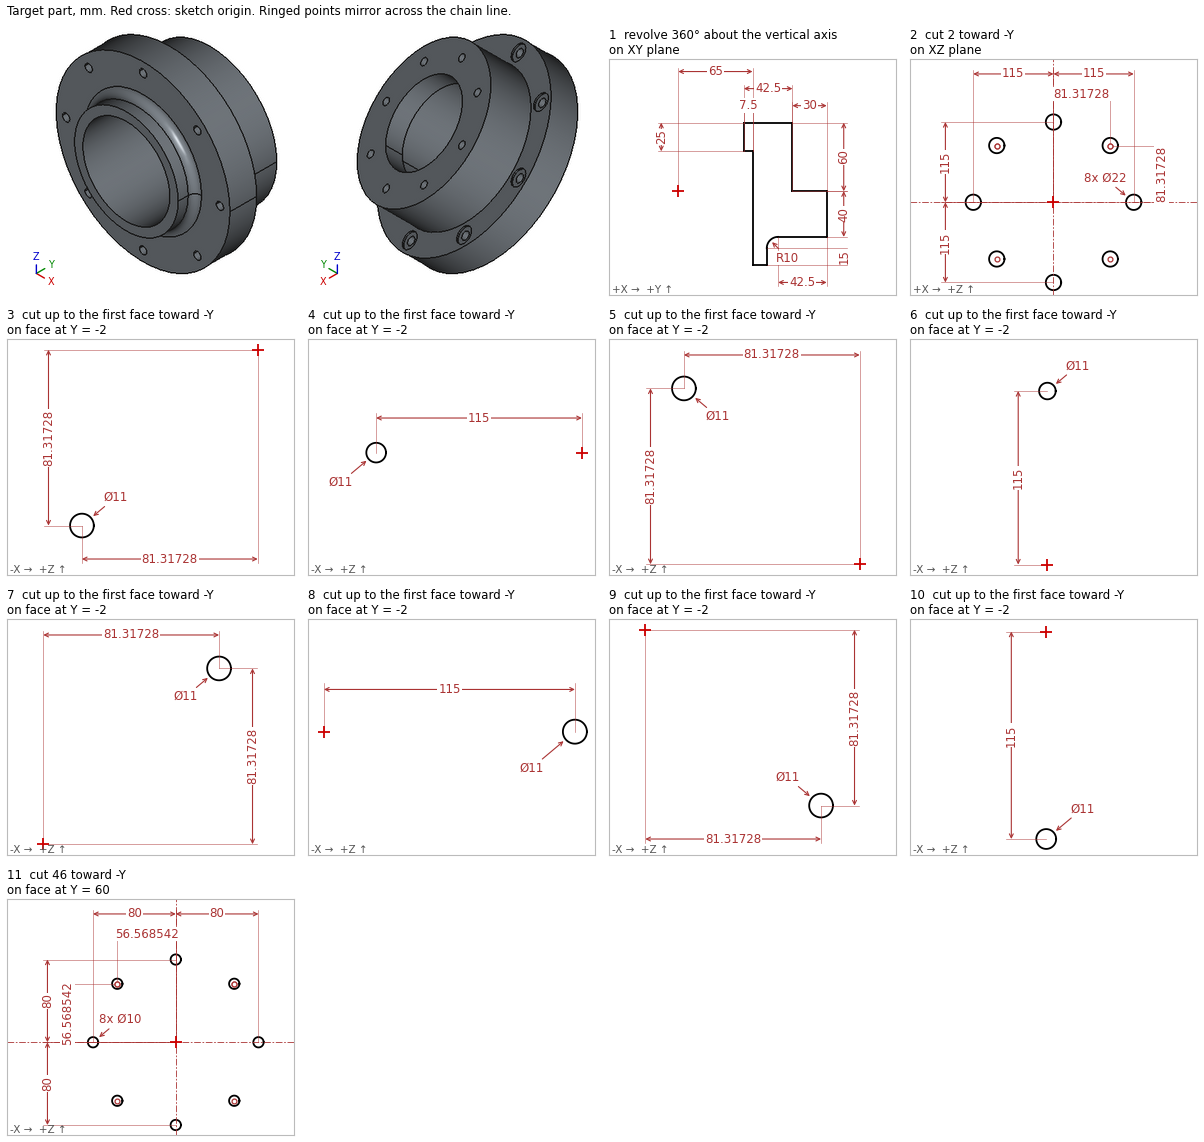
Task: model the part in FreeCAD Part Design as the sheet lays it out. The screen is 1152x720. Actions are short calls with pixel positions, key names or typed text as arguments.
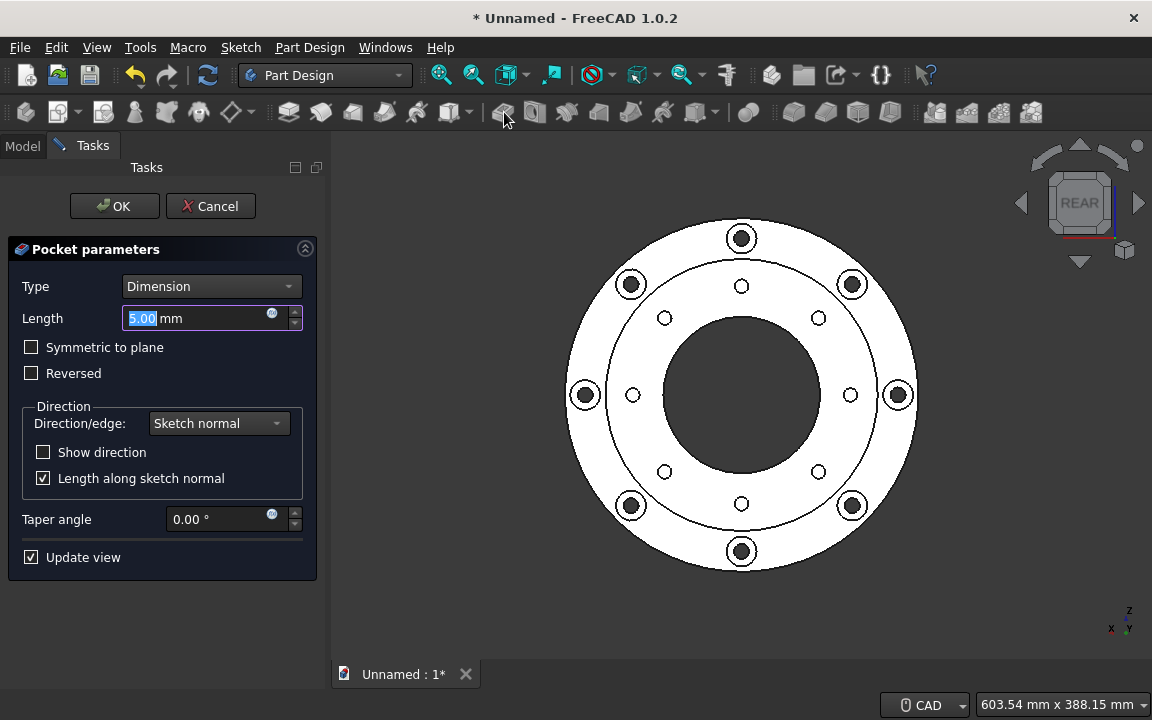
text(46)
key(Tab)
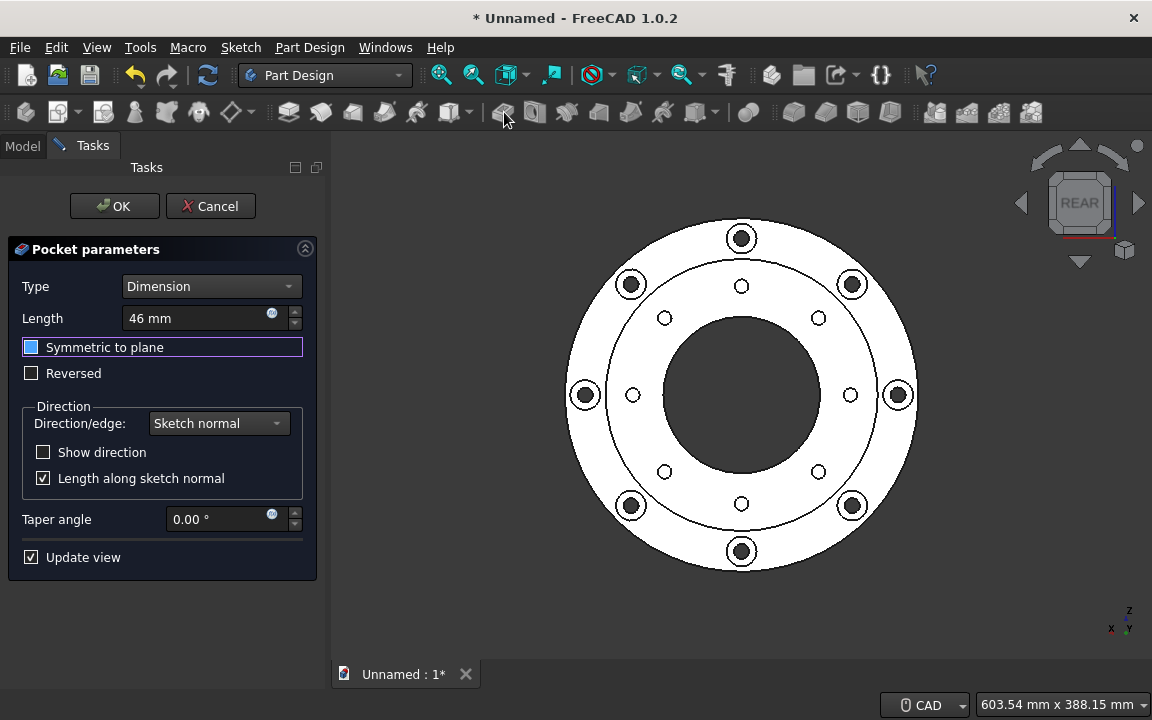
click(115, 206)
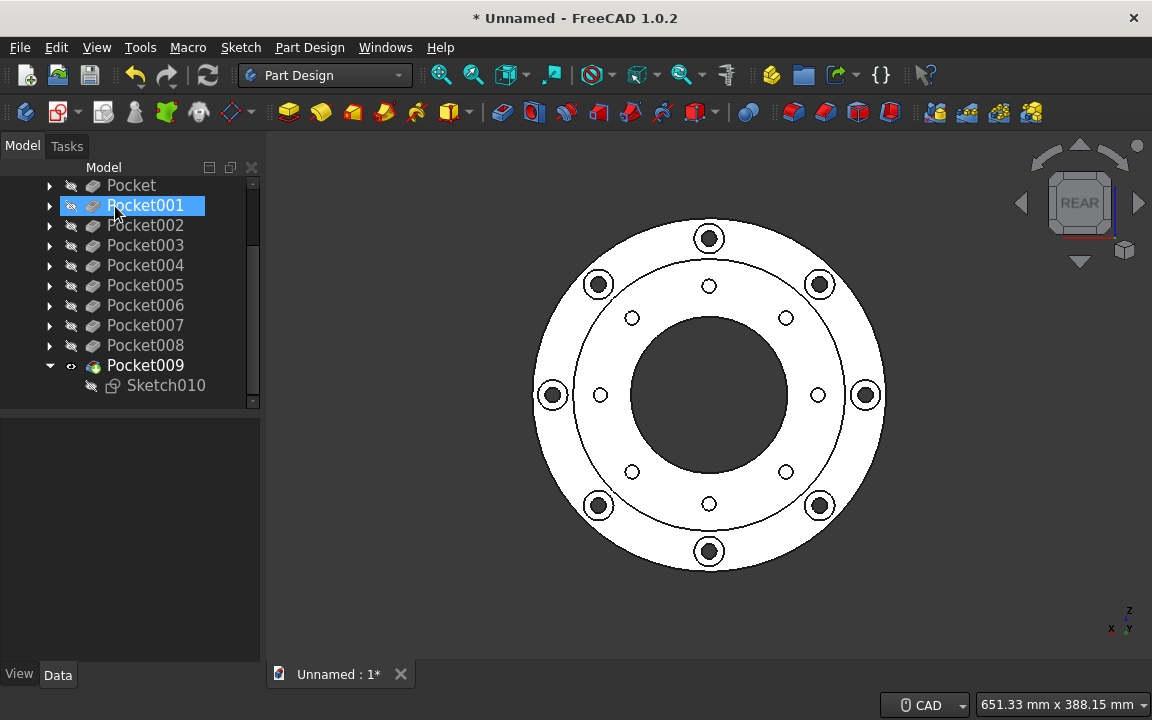
key(0)